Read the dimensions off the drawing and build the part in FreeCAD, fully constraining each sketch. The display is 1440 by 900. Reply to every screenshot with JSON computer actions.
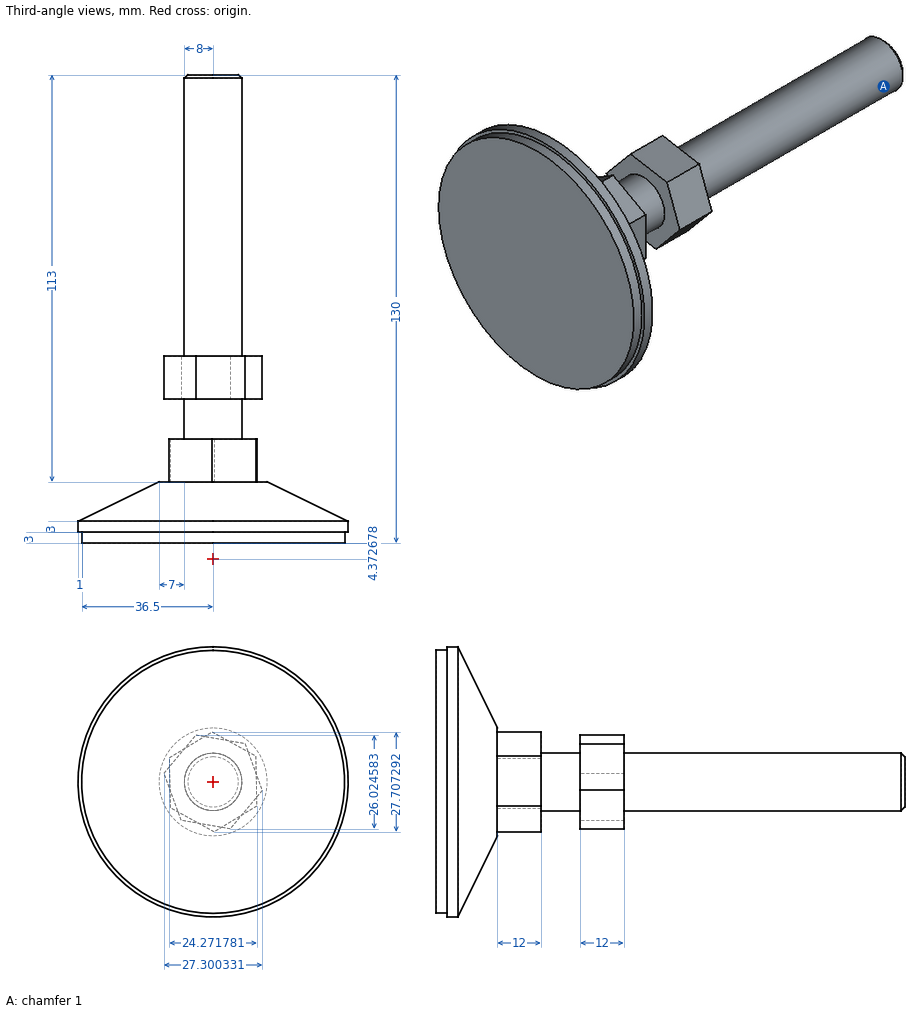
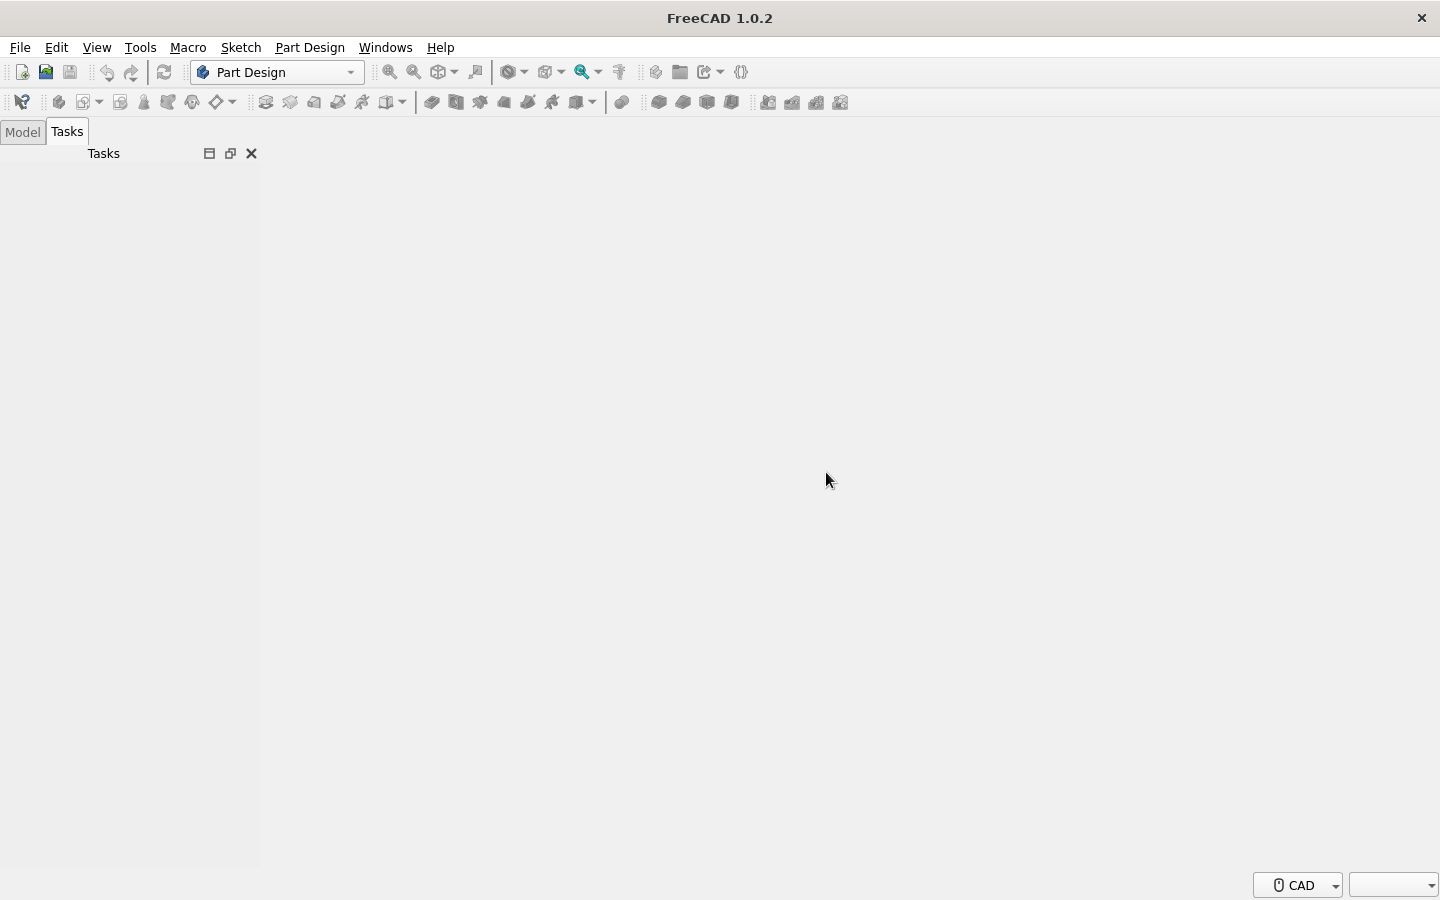
{"action": "left_click", "coordinate": [22, 72]}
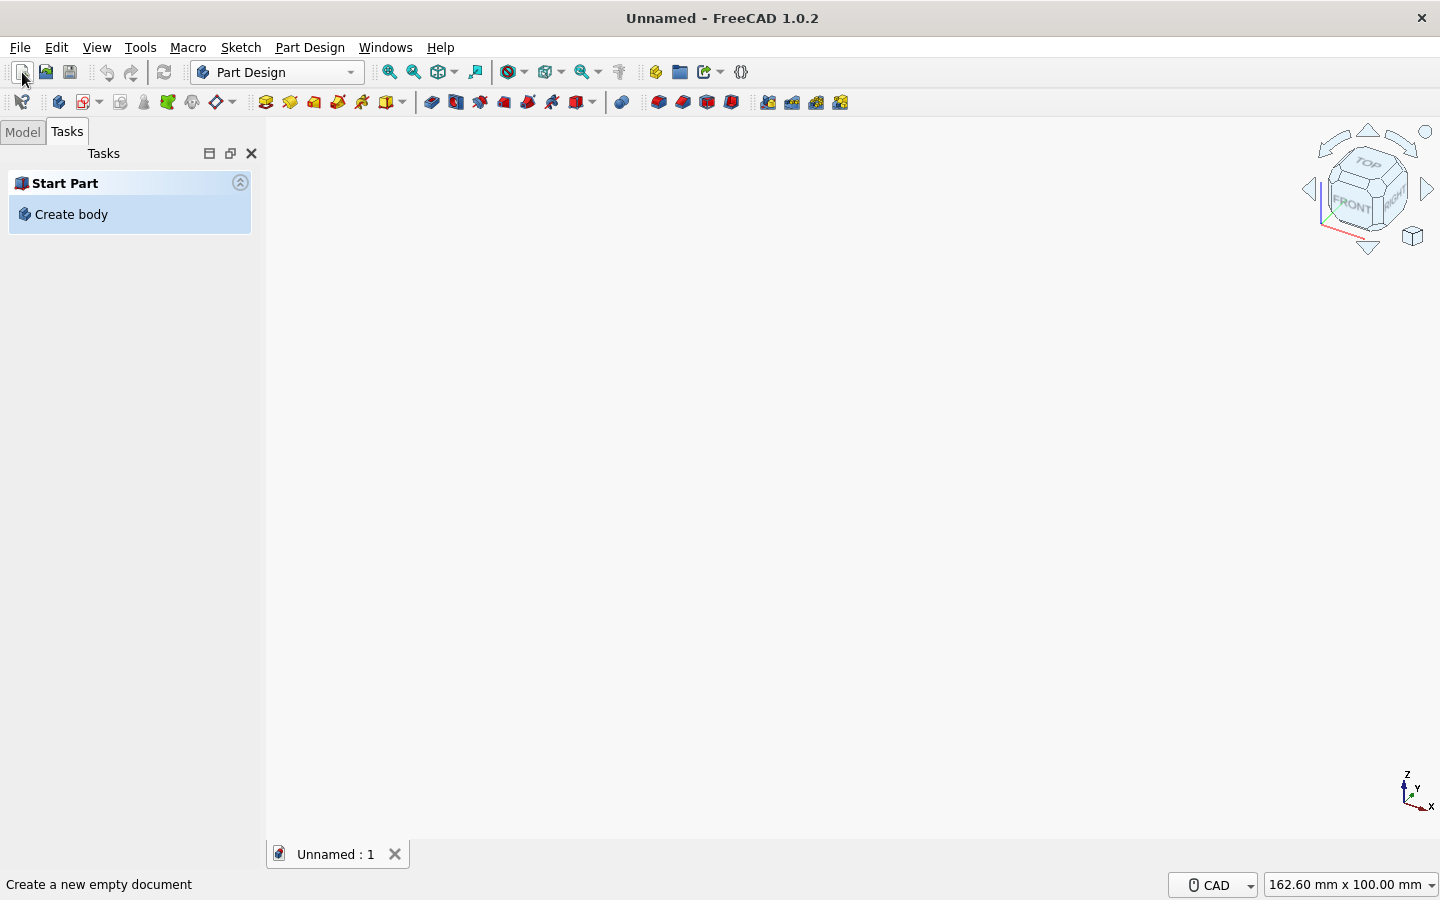
{"action": "left_click", "coordinate": [84, 102]}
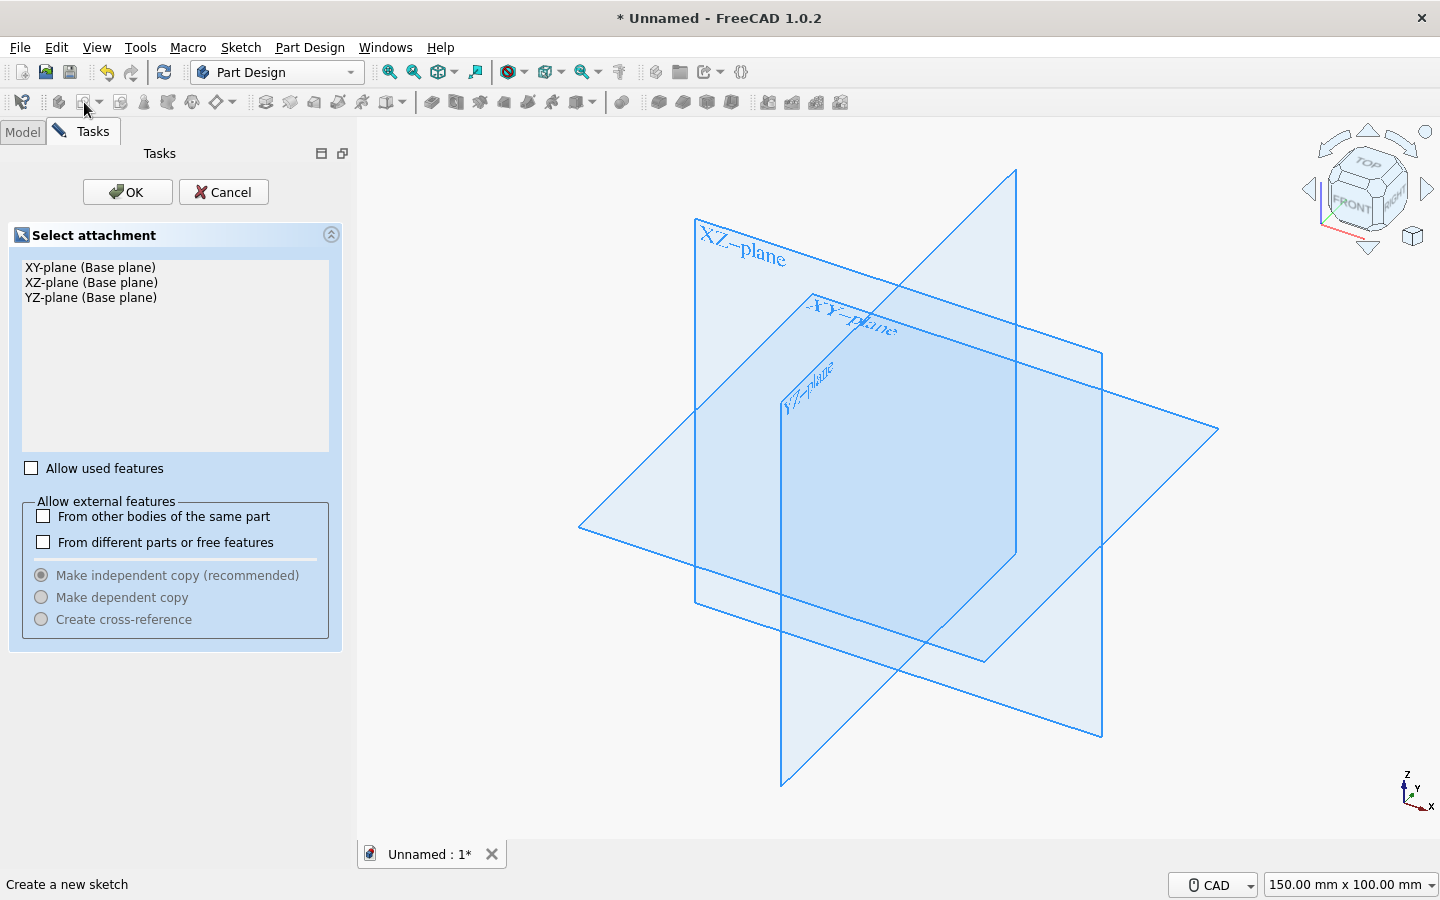
{"action": "left_click", "coordinate": [82, 268]}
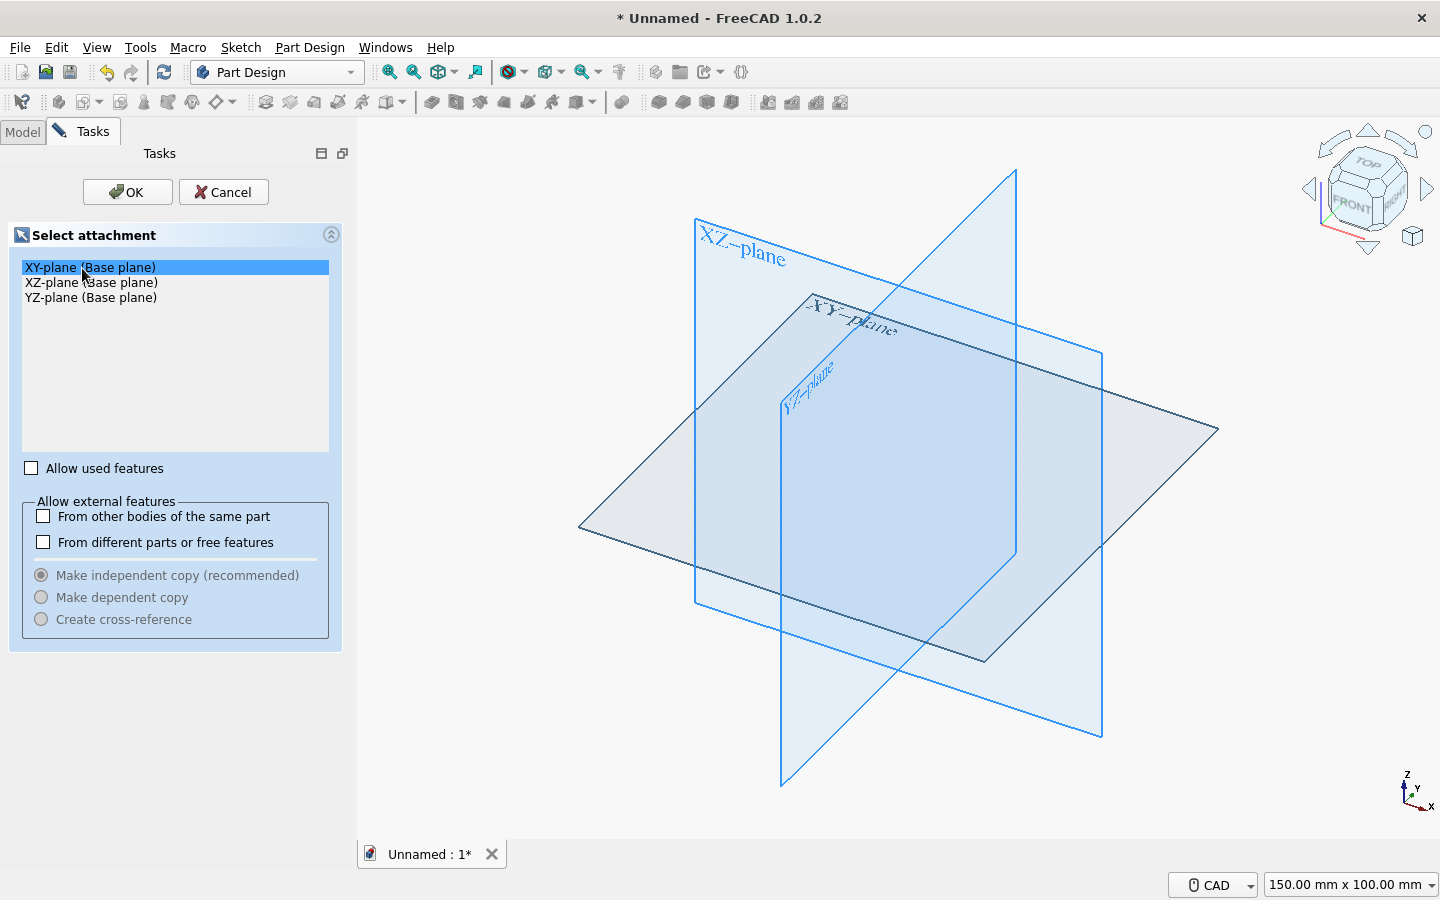
{"action": "left_click", "coordinate": [128, 192]}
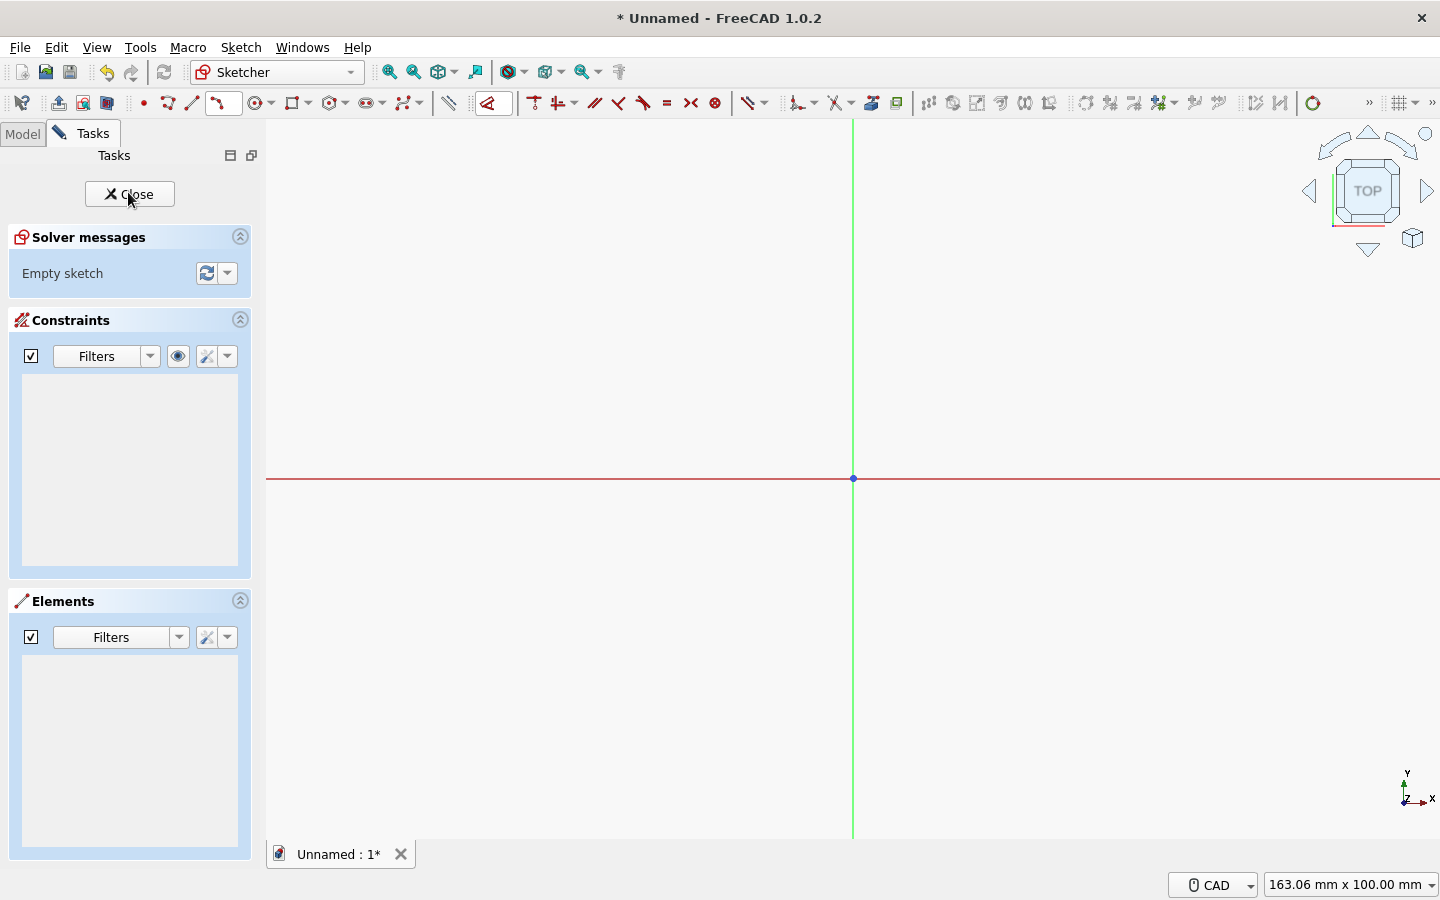
{"action": "scroll", "coordinate": [839, 811], "scroll_direction": "down", "scroll_amount": 4}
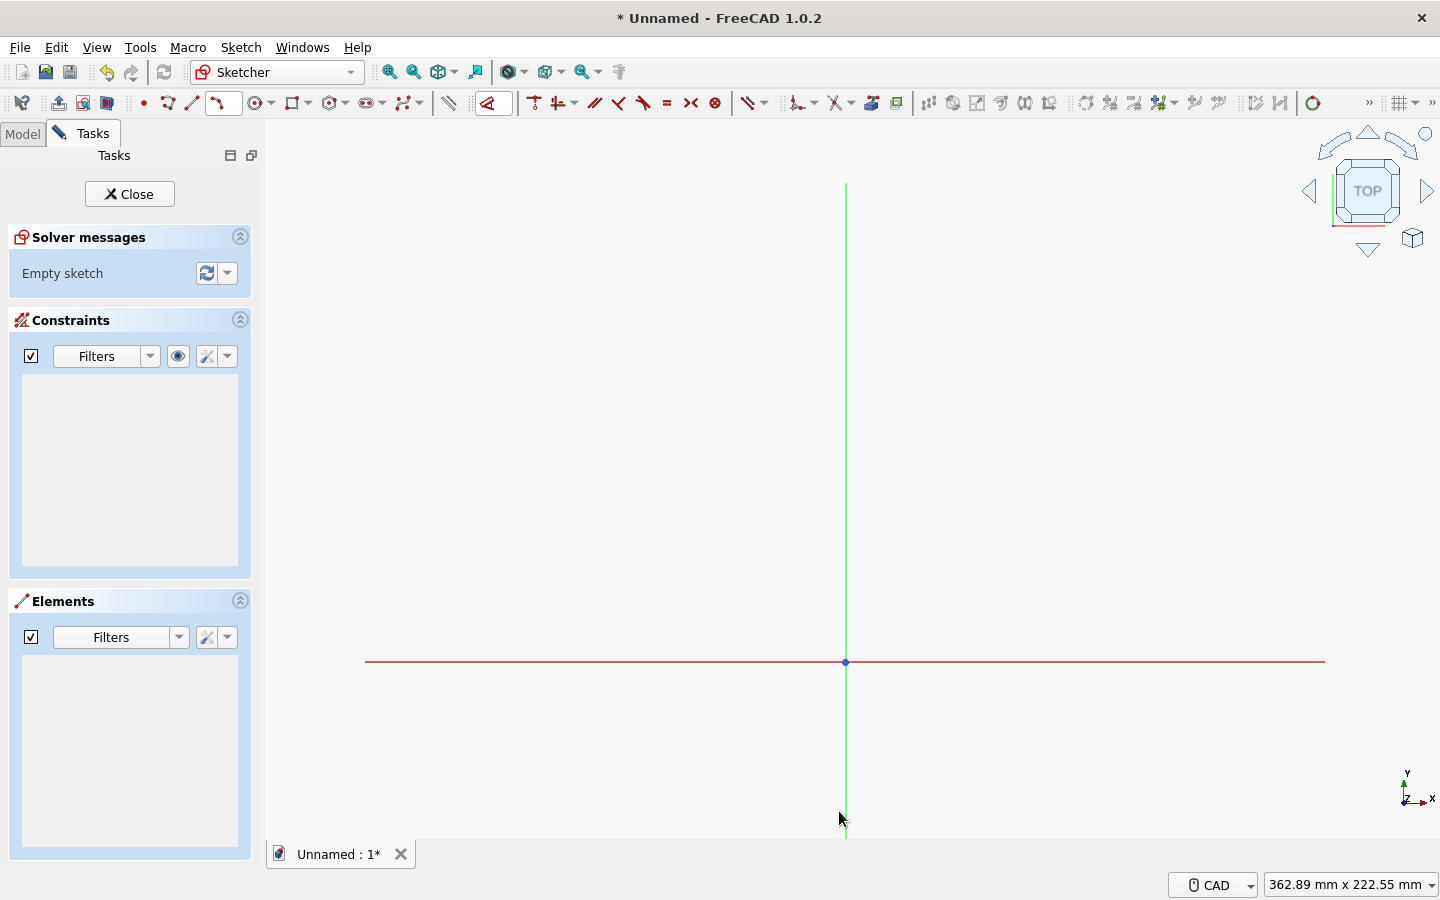
{"action": "left_click", "coordinate": [168, 104]}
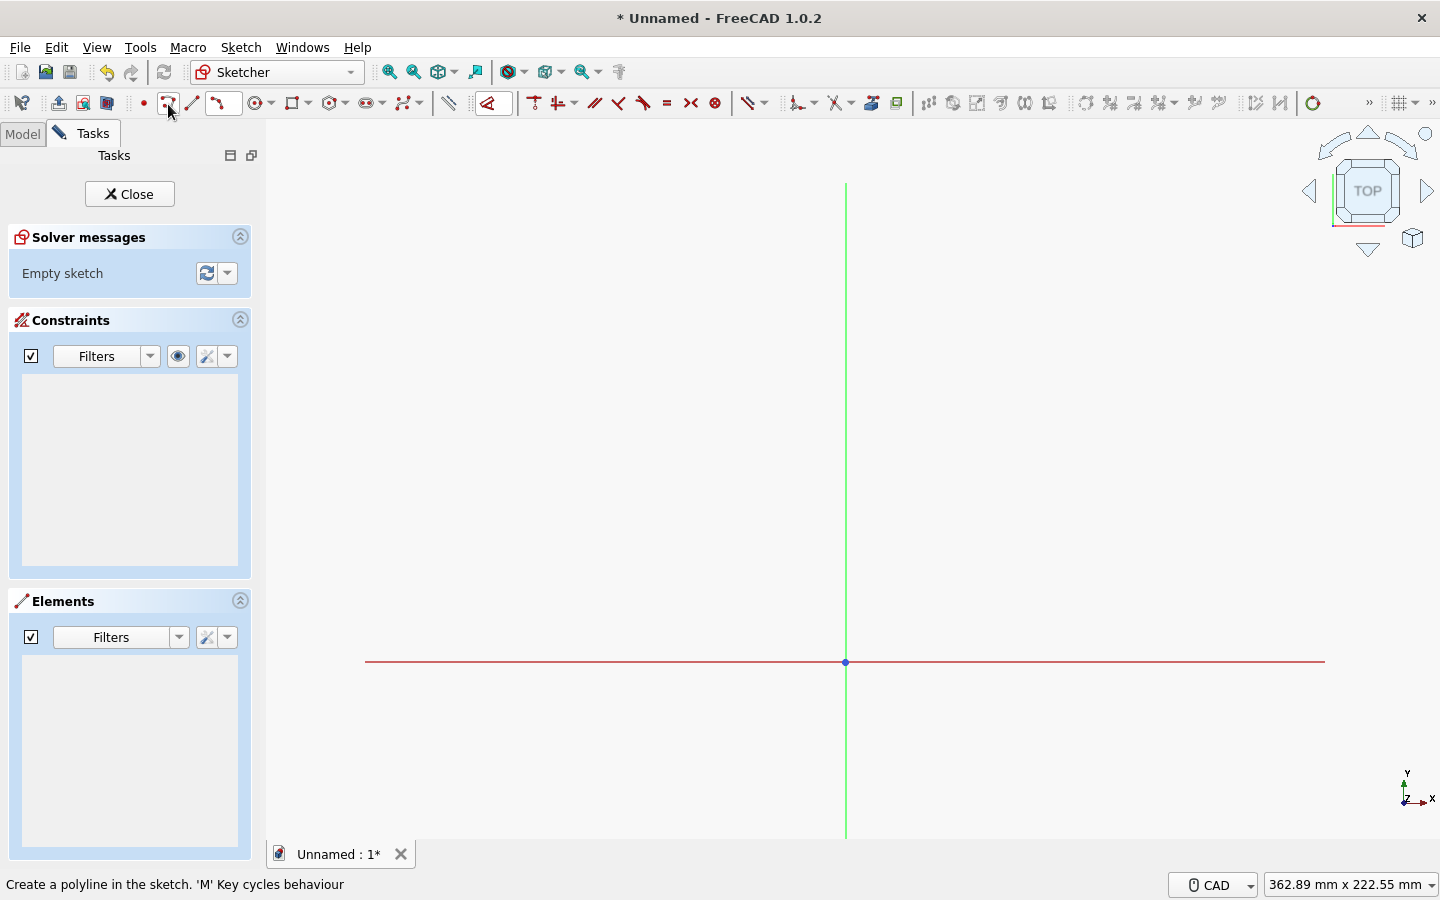
{"action": "left_click", "coordinate": [846, 648]}
{"action": "left_click", "coordinate": [837, 228]}
{"action": "left_click", "coordinate": [820, 228]}
{"action": "left_click", "coordinate": [820, 593]}
{"action": "left_click", "coordinate": [797, 593]}
{"action": "left_click", "coordinate": [724, 629]}